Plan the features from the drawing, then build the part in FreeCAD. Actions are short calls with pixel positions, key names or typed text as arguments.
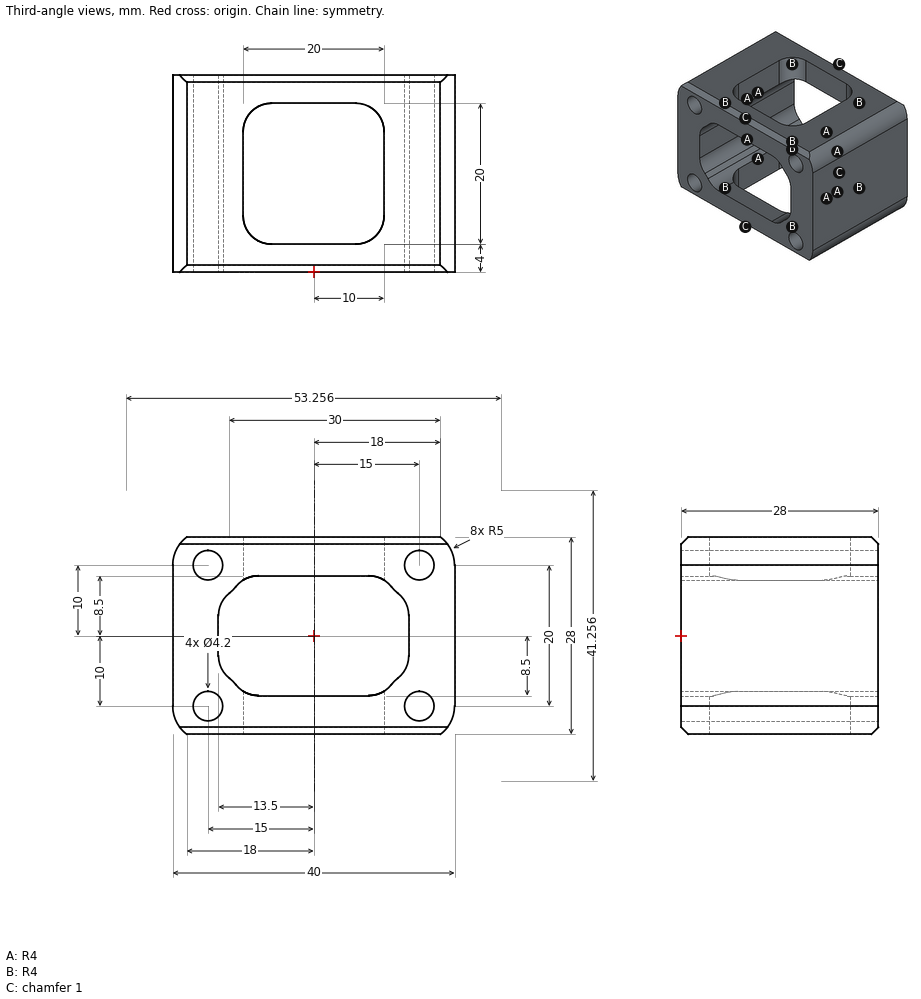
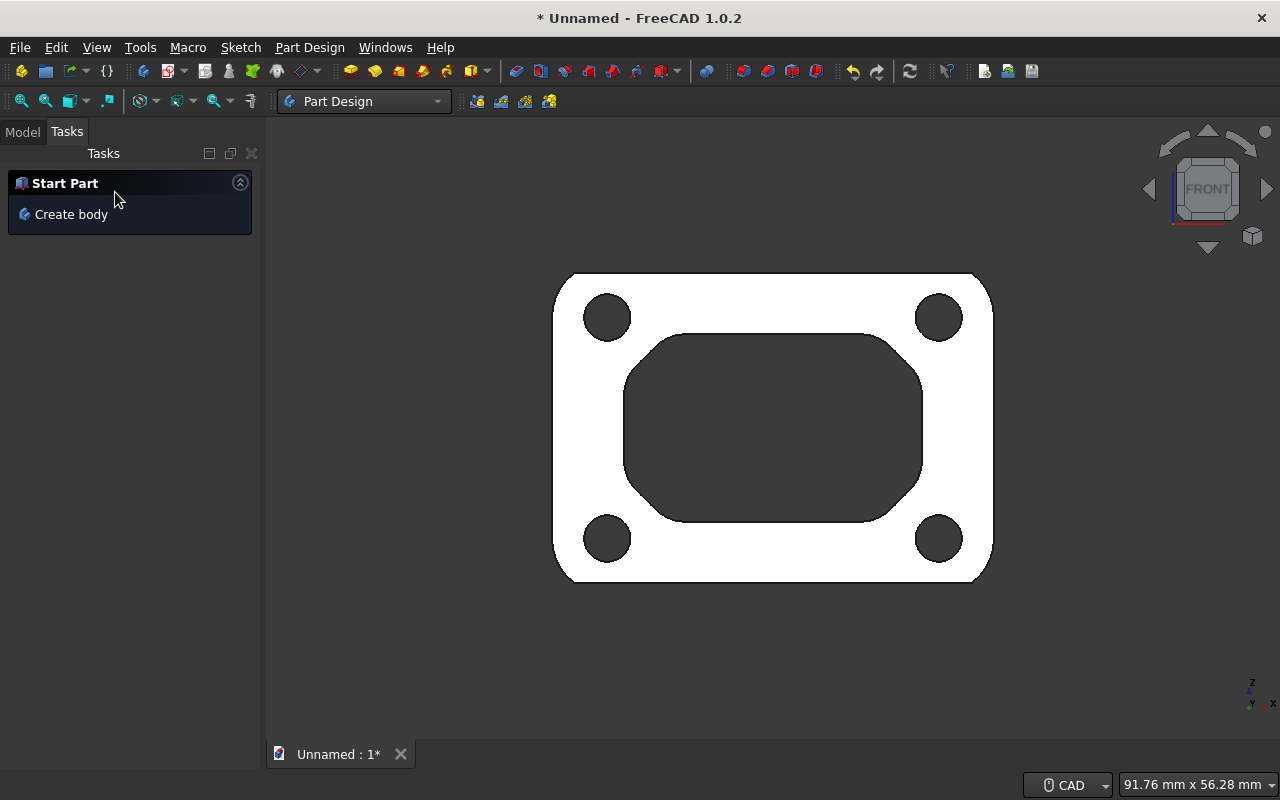
key(3)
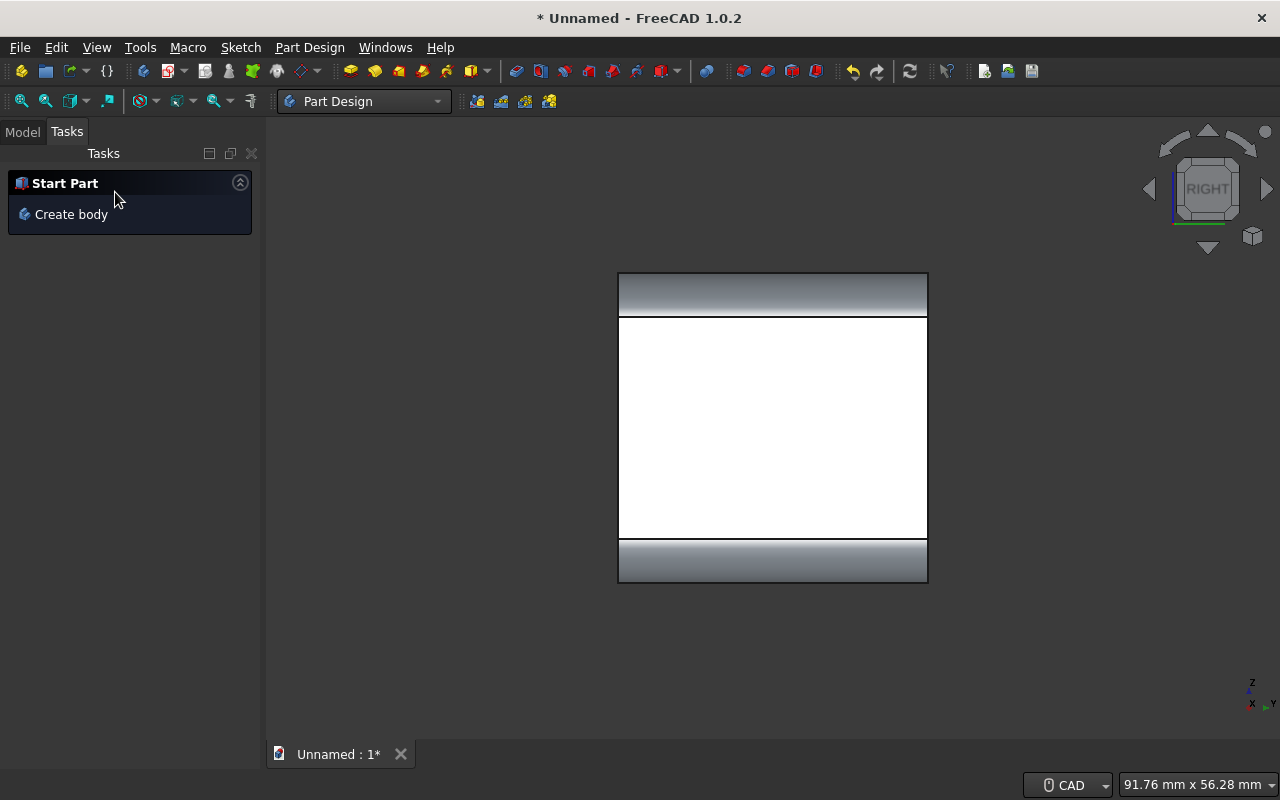
key(5)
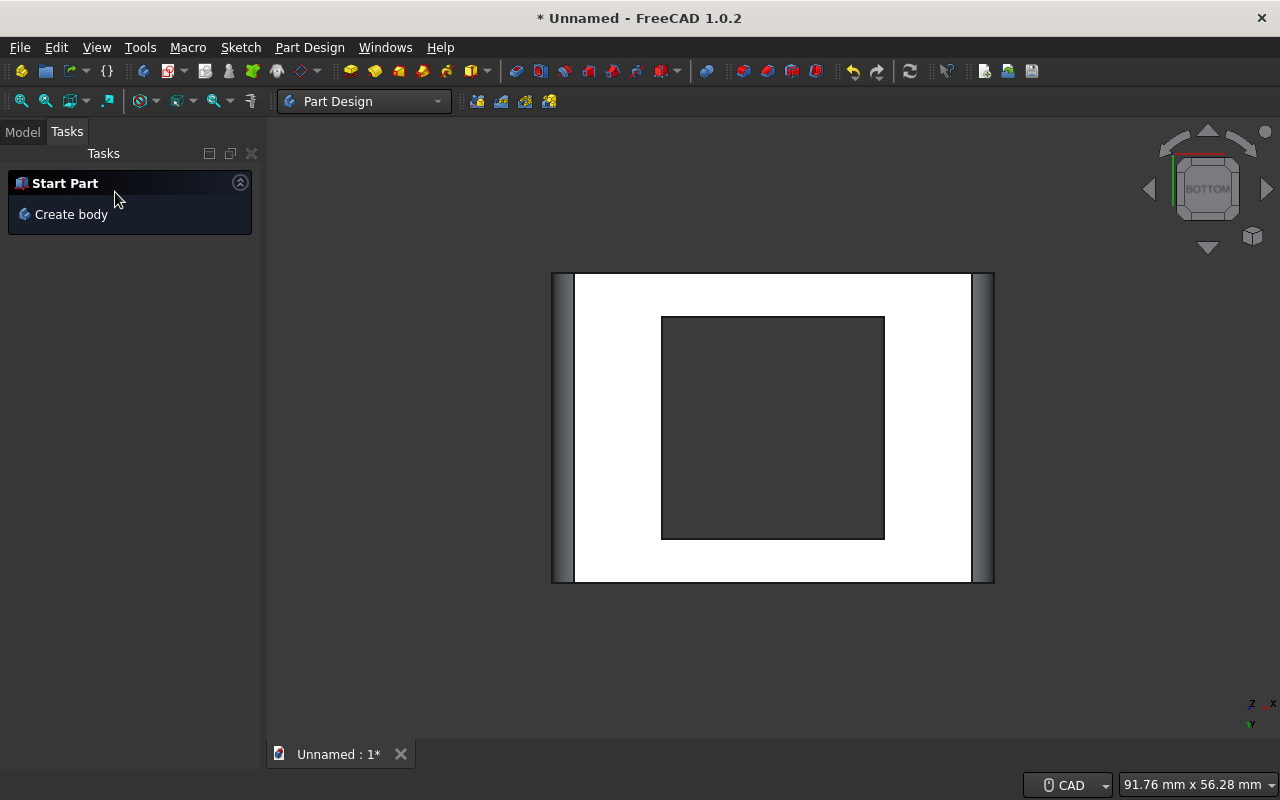
key(4)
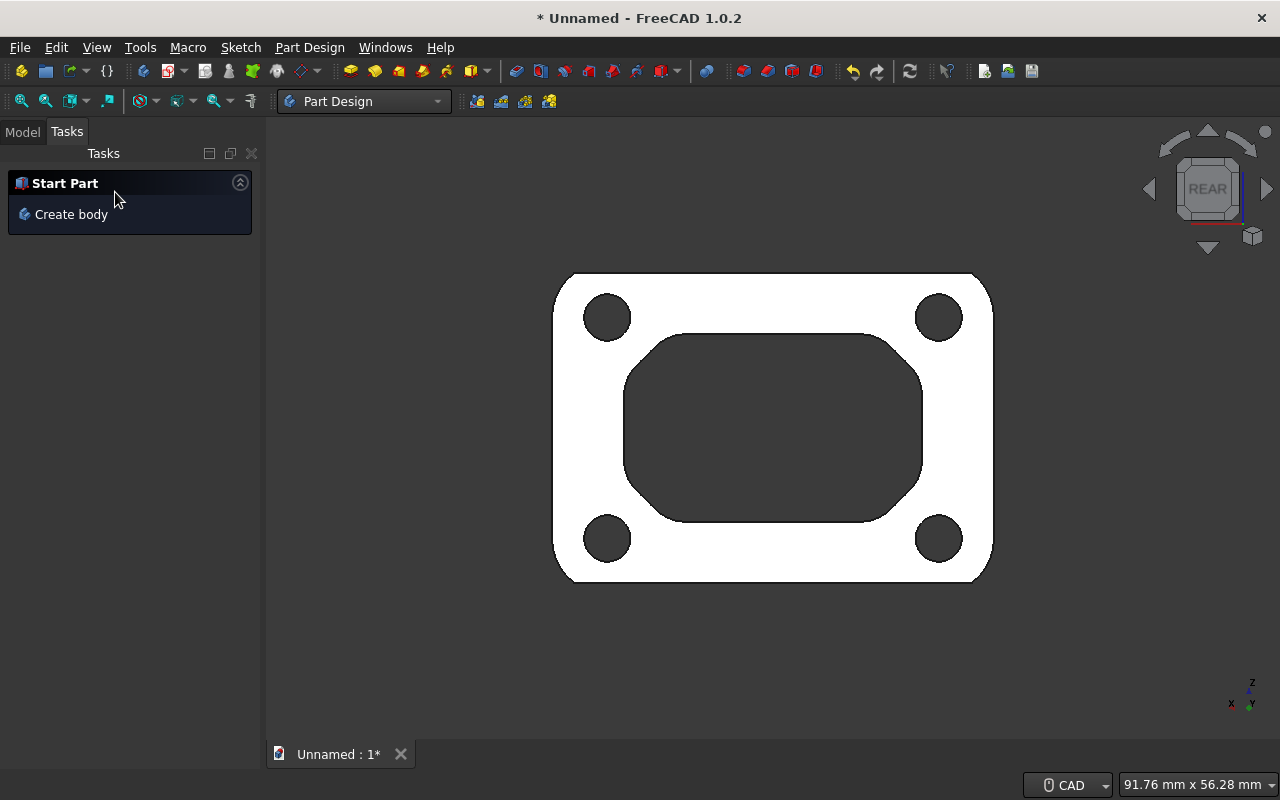
key(6)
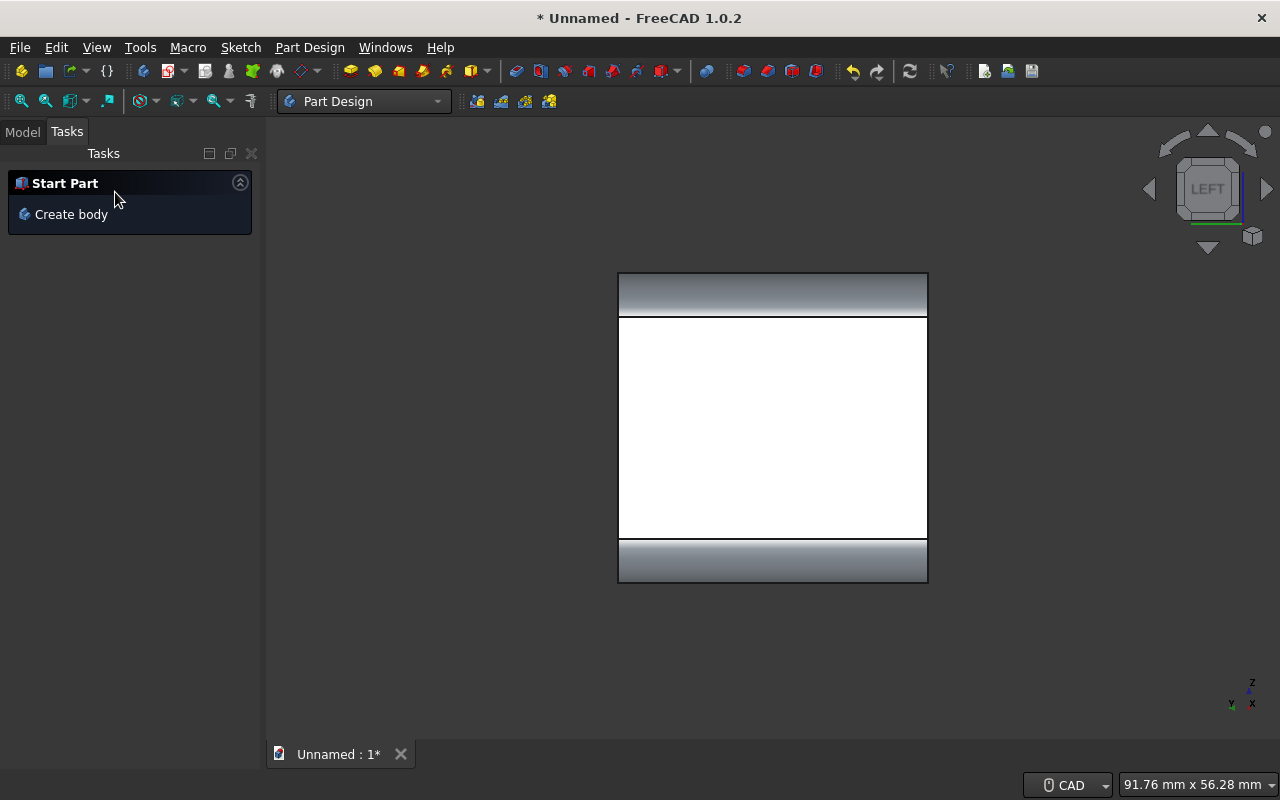
key(v)
key(3)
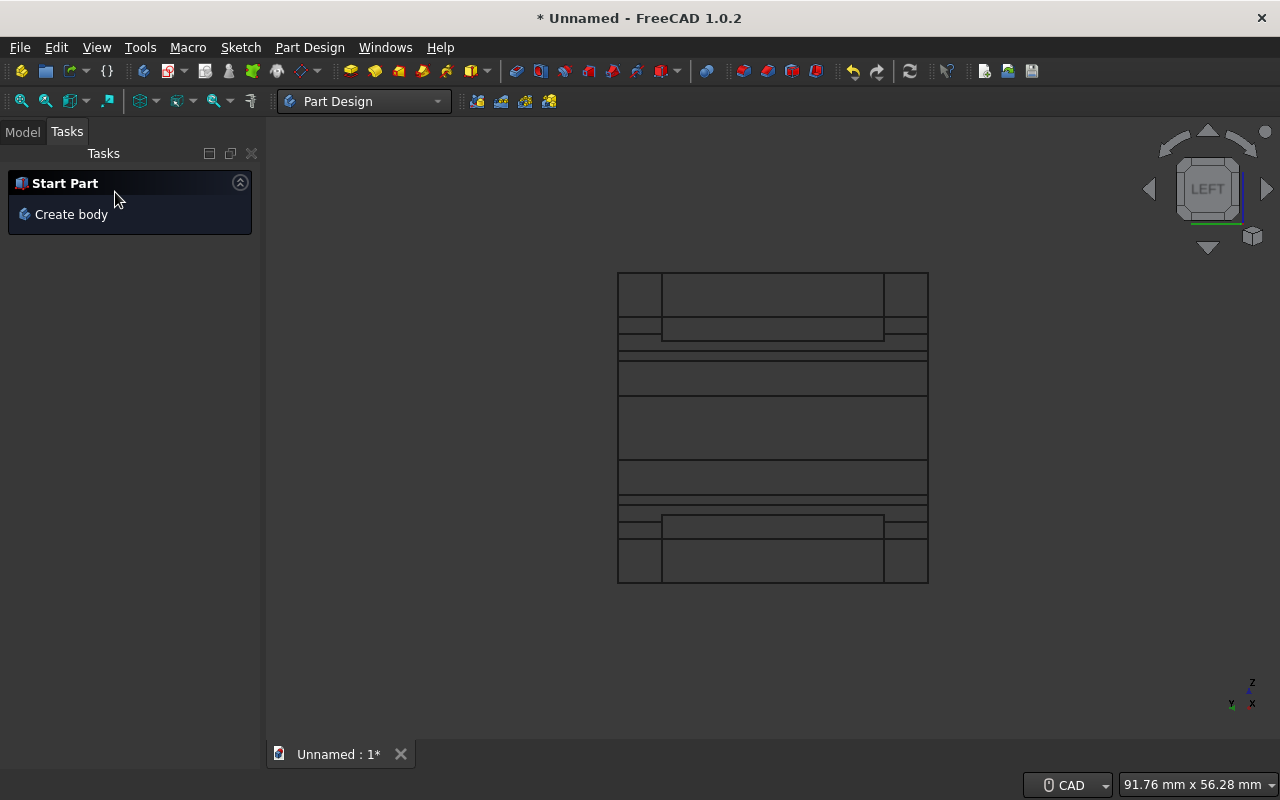
key(0)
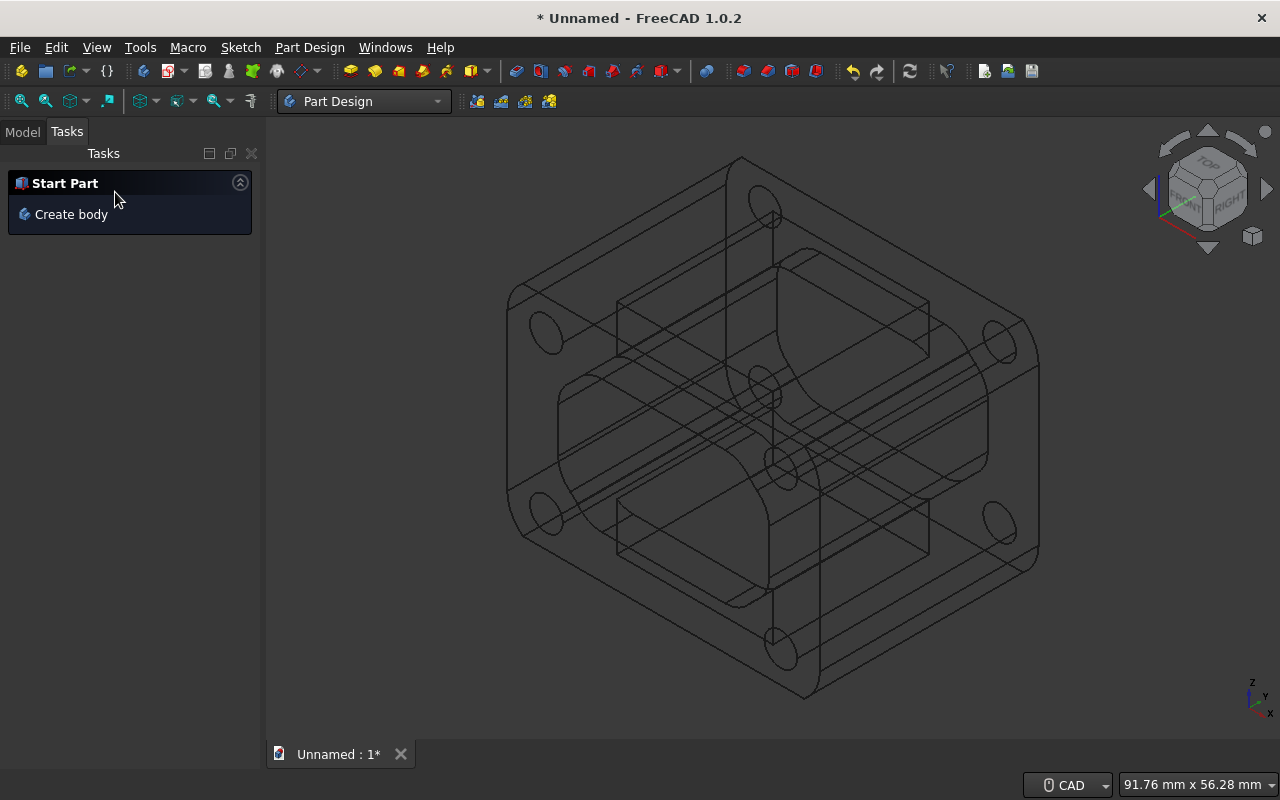
click(773, 616)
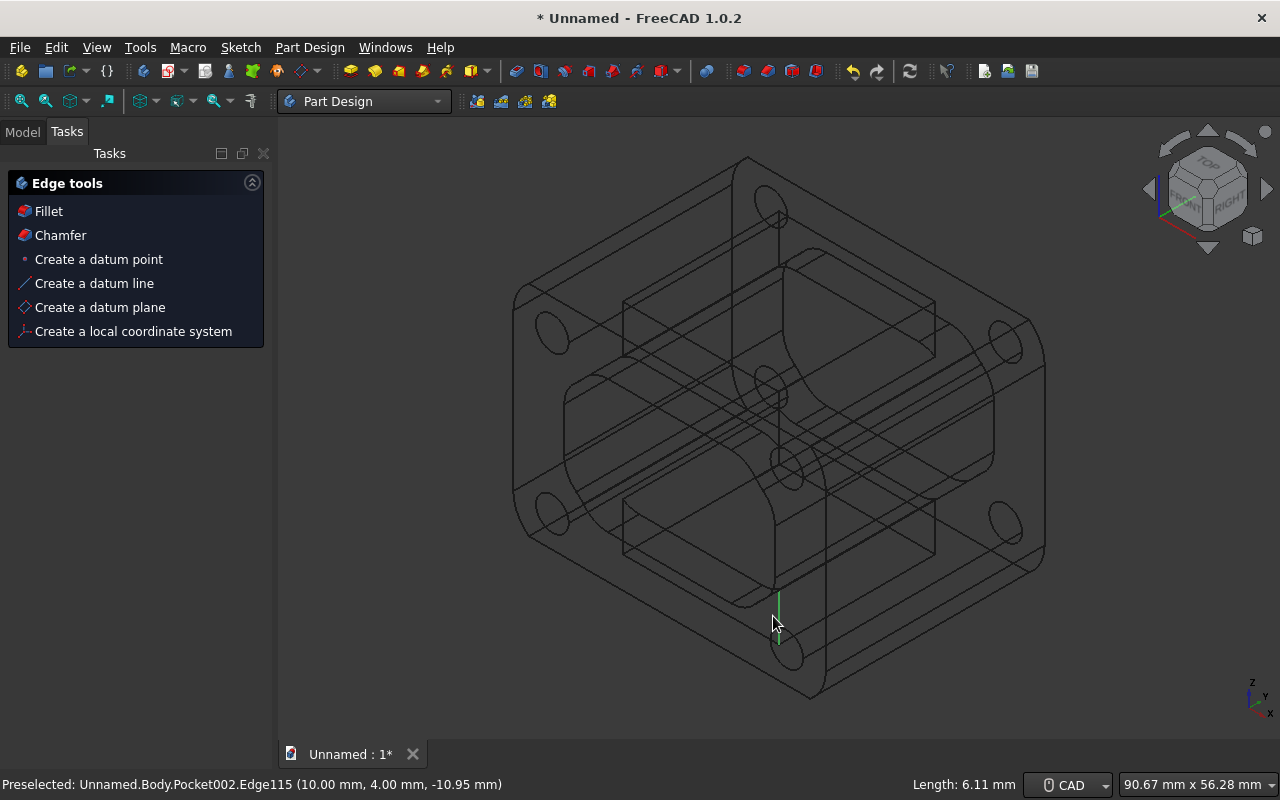
click(623, 531, ctrl)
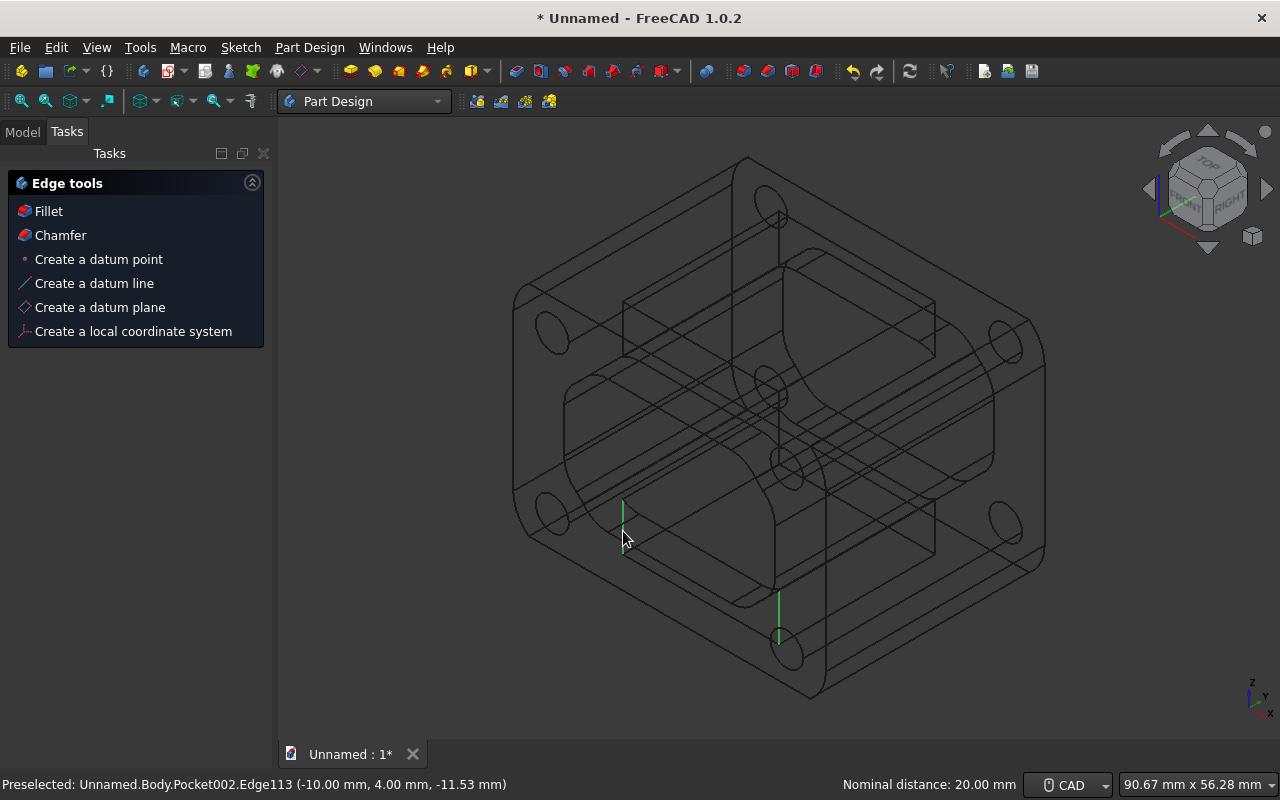
click(779, 456, ctrl)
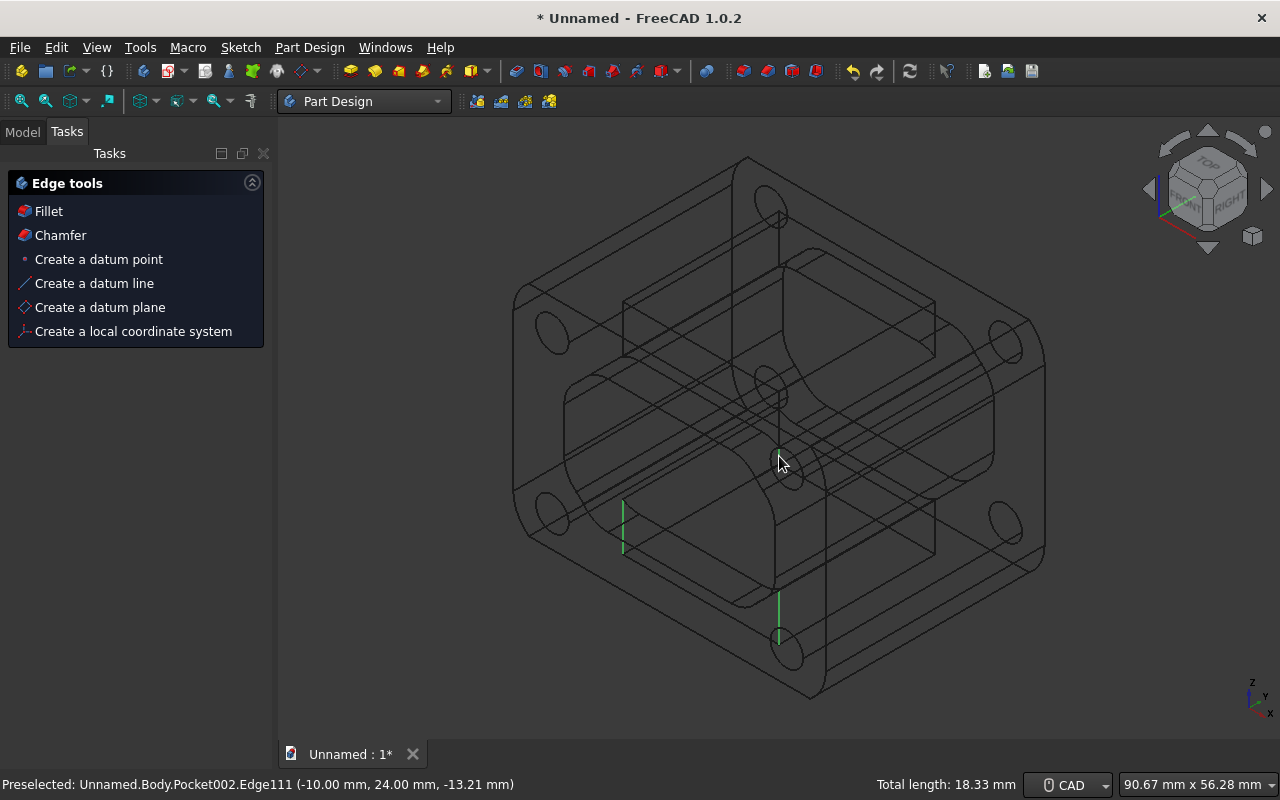
click(935, 526, ctrl)